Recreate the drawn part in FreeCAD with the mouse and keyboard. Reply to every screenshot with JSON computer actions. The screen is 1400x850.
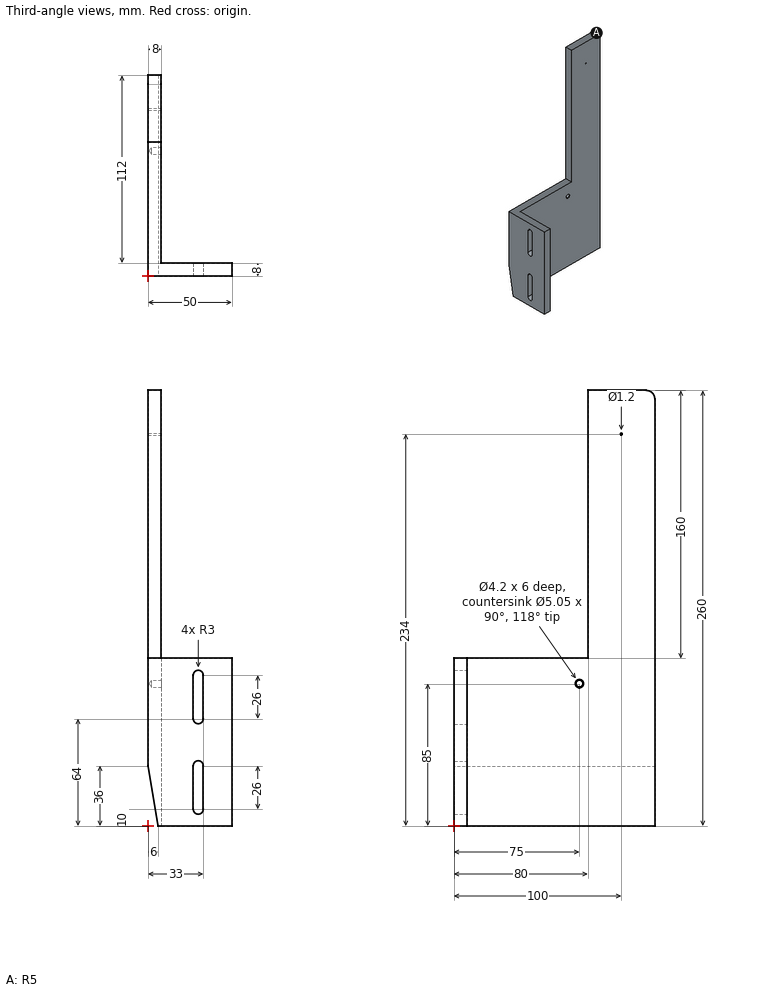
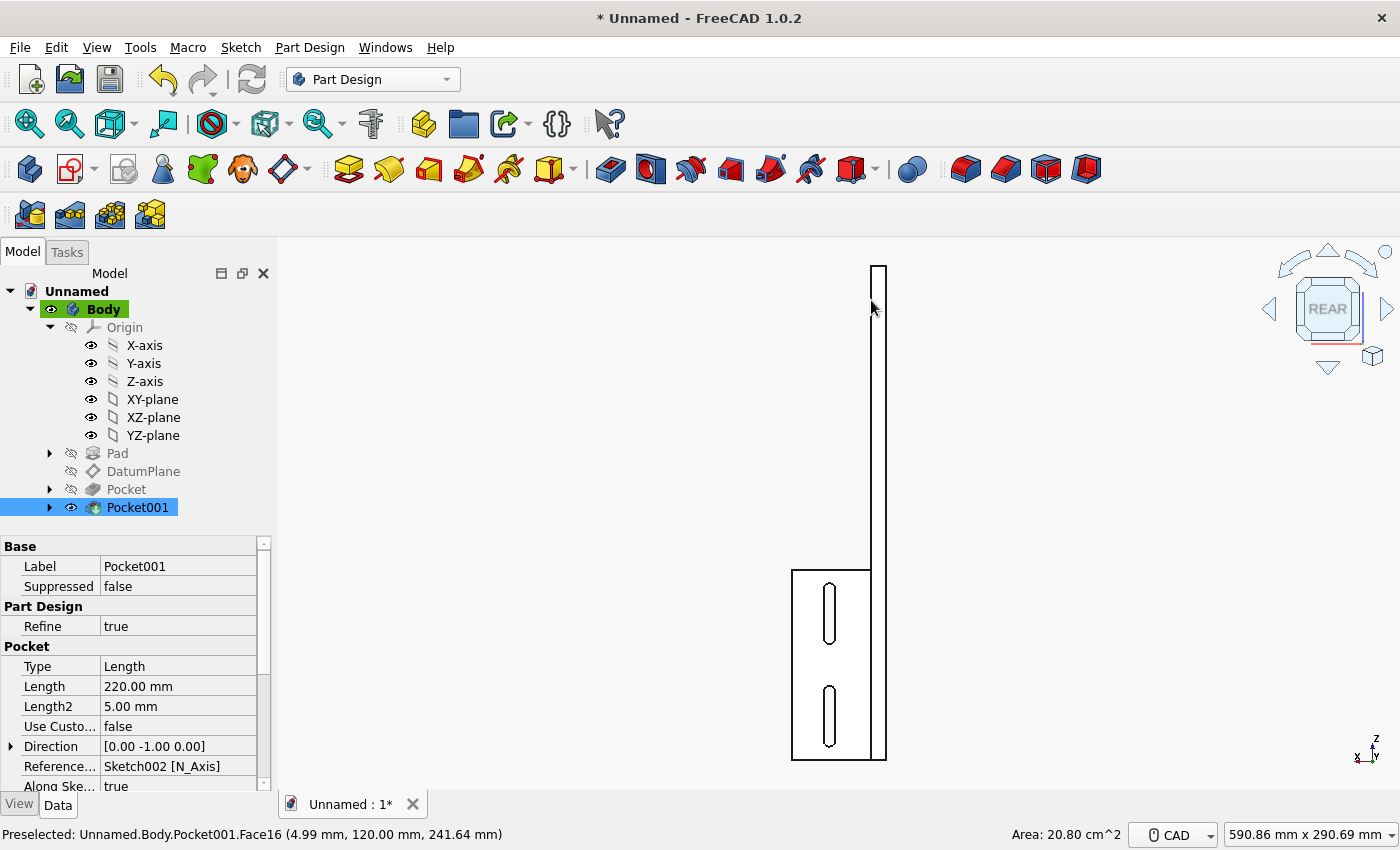
{"action": "left_click", "coordinate": [70, 170]}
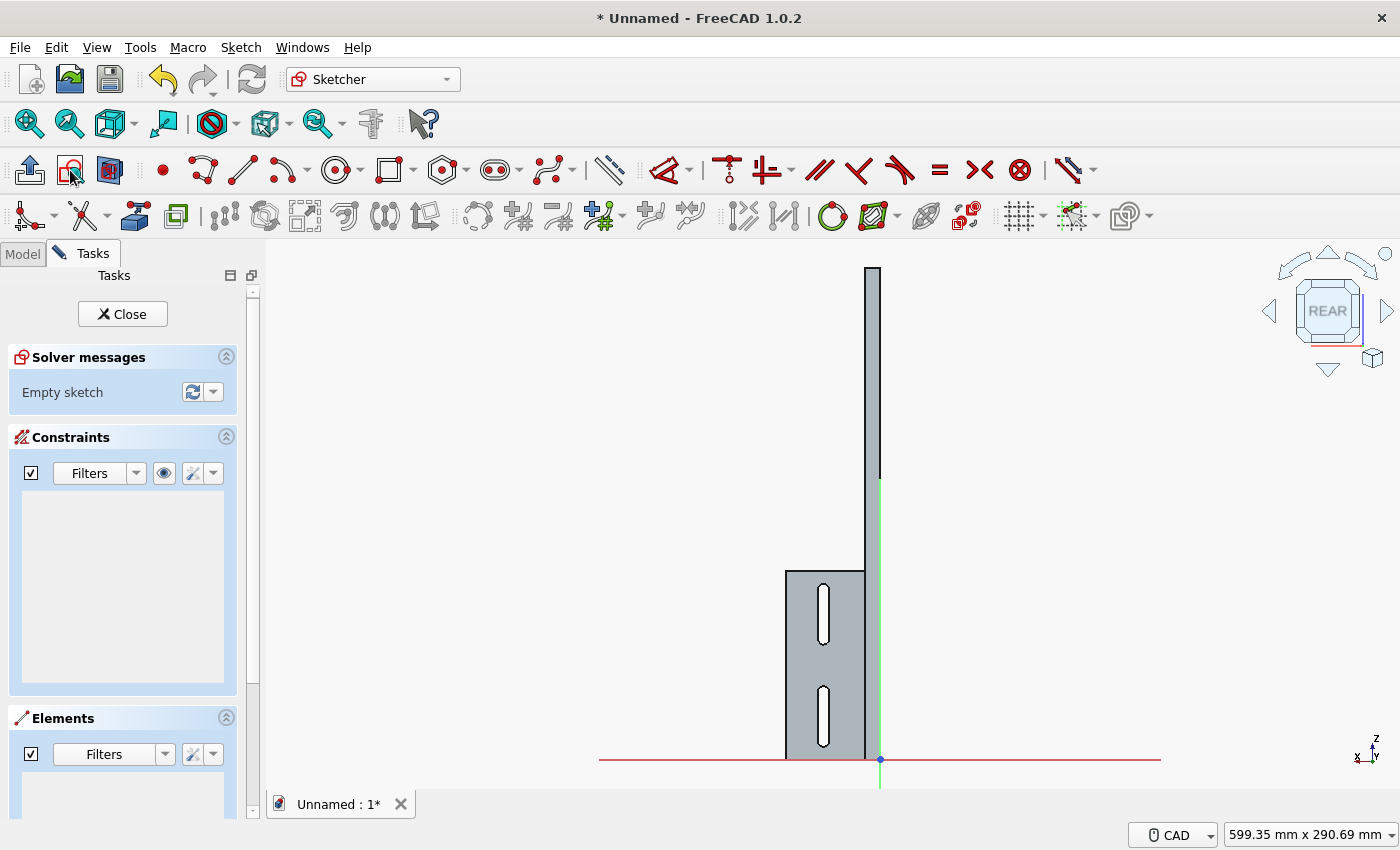
{"action": "scroll", "coordinate": [764, 514], "scroll_direction": "down", "scroll_amount": 5}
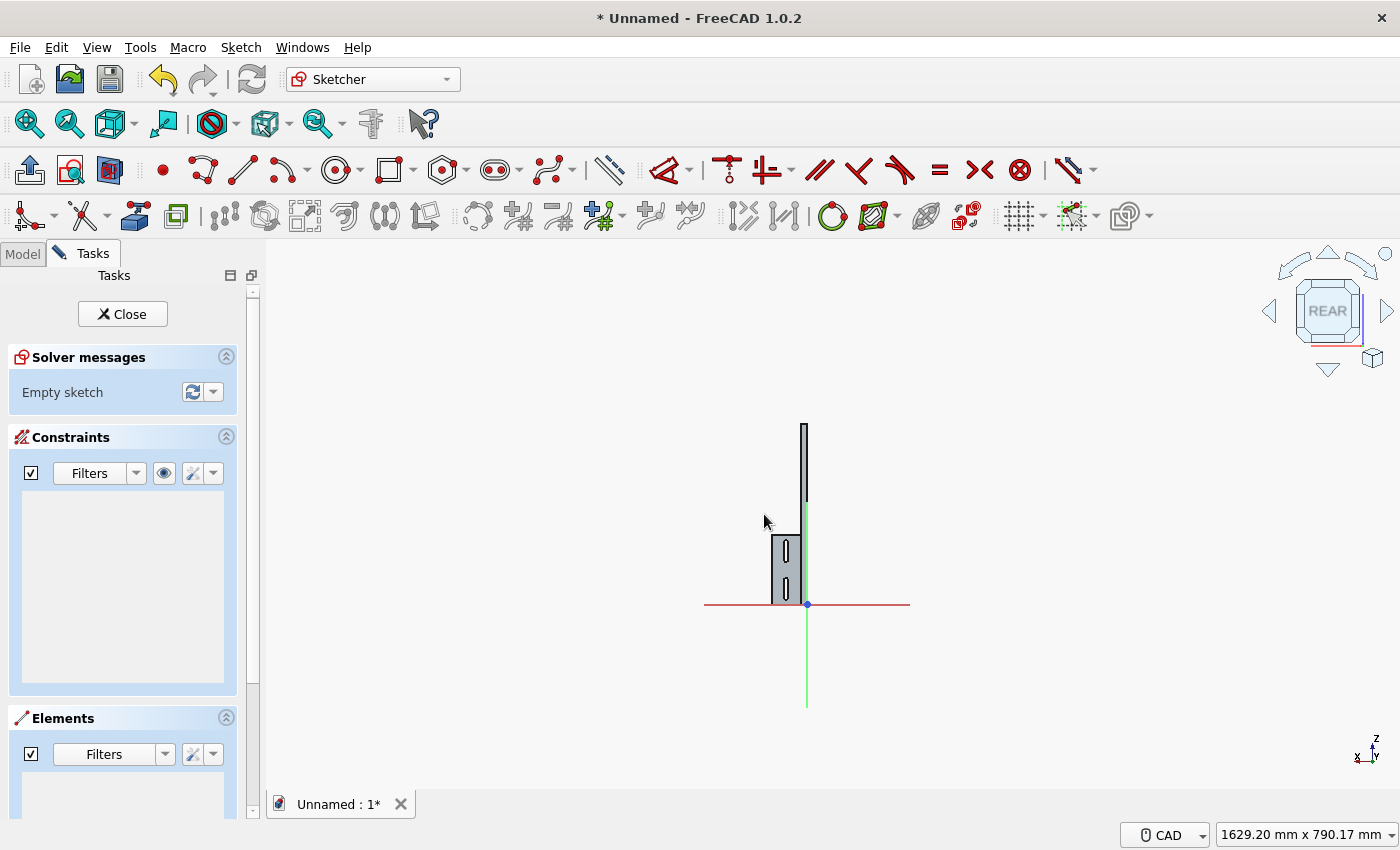
{"action": "scroll", "coordinate": [808, 599], "scroll_direction": "up", "scroll_amount": 13}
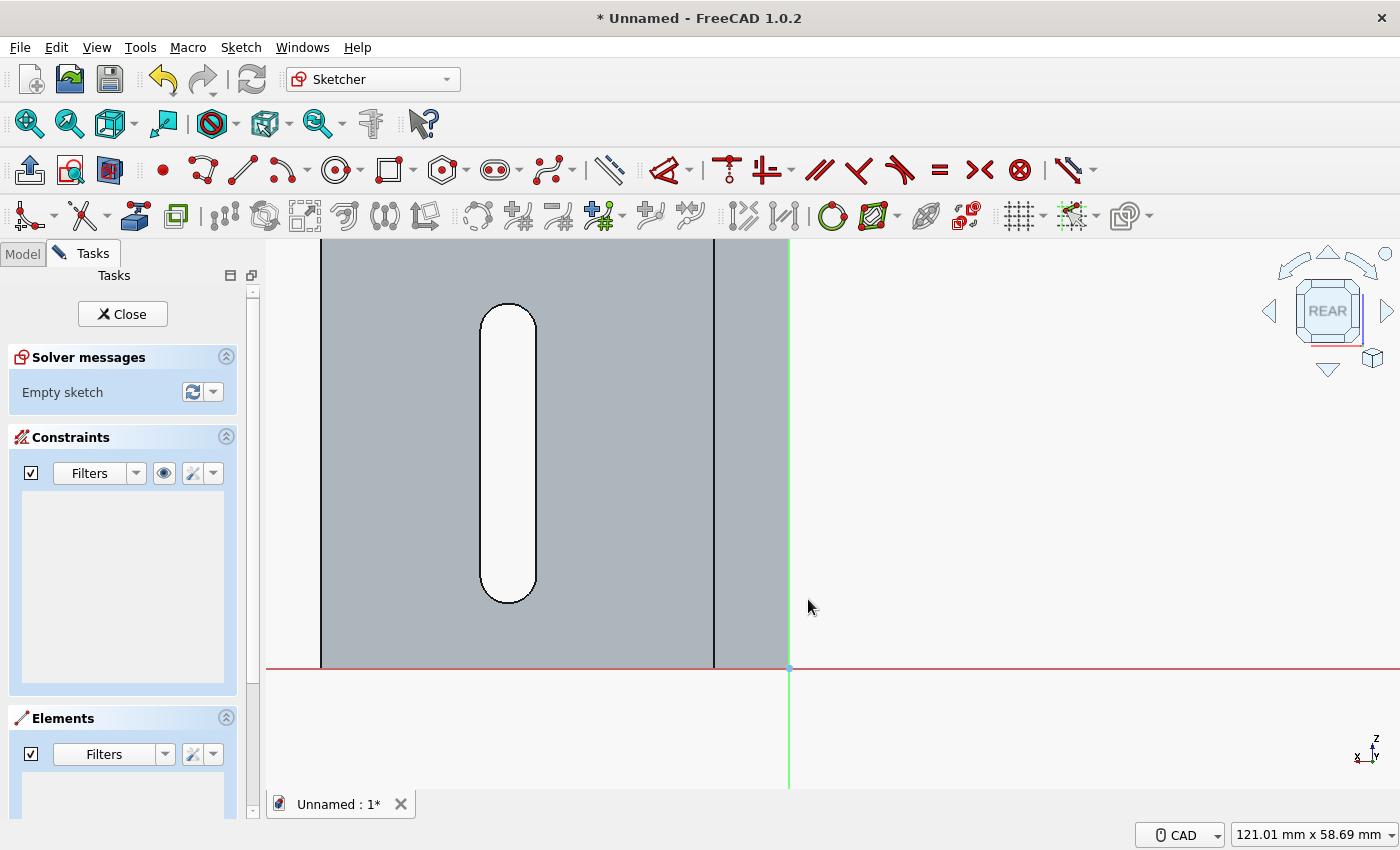
{"action": "left_click", "coordinate": [204, 170]}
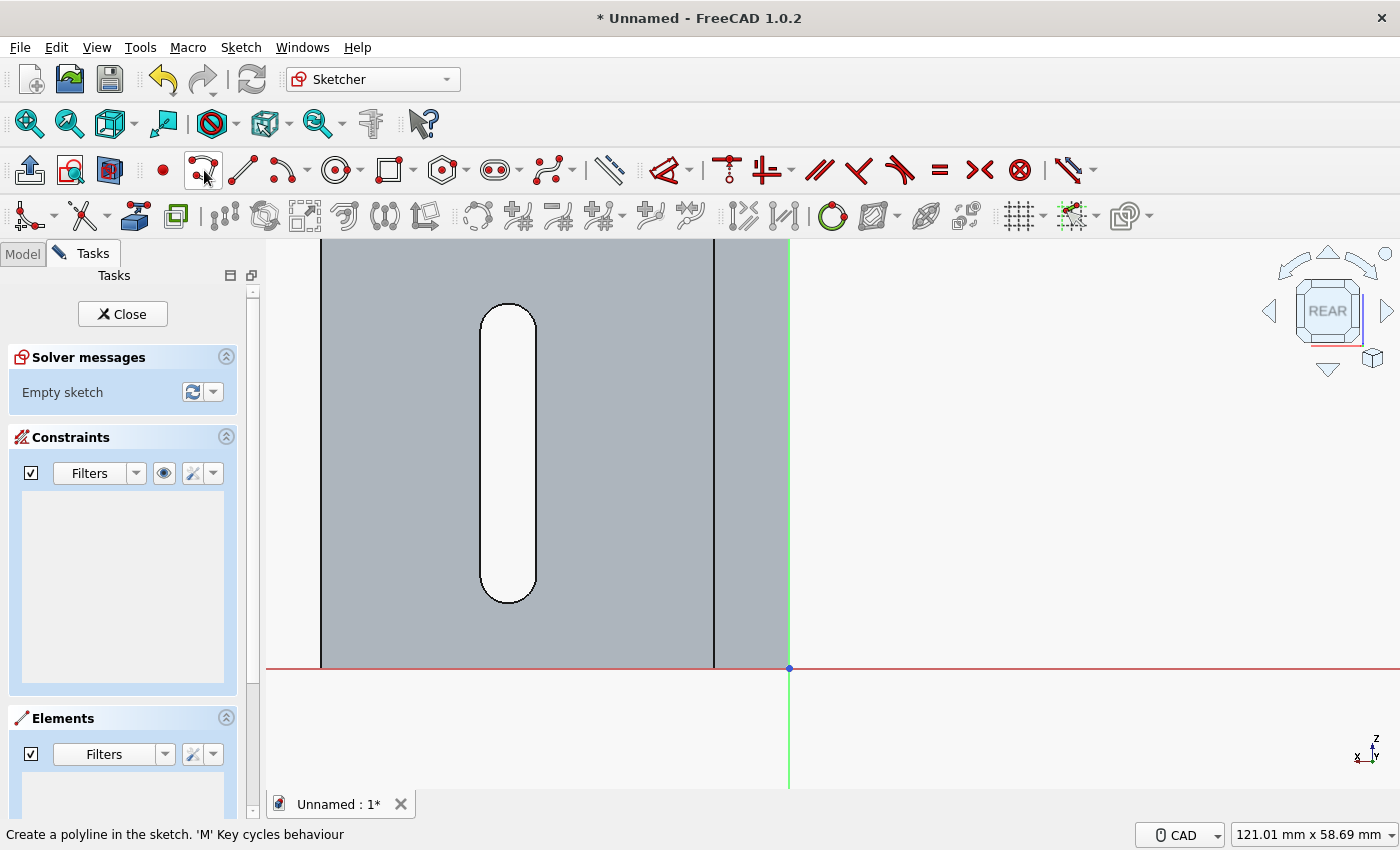
{"action": "left_click", "coordinate": [789, 669]}
{"action": "left_click", "coordinate": [780, 332]}
{"action": "left_click", "coordinate": [733, 660]}
{"action": "left_click", "coordinate": [789, 669]}
{"action": "key", "text": "Escape"}
{"action": "key", "text": "Escape"}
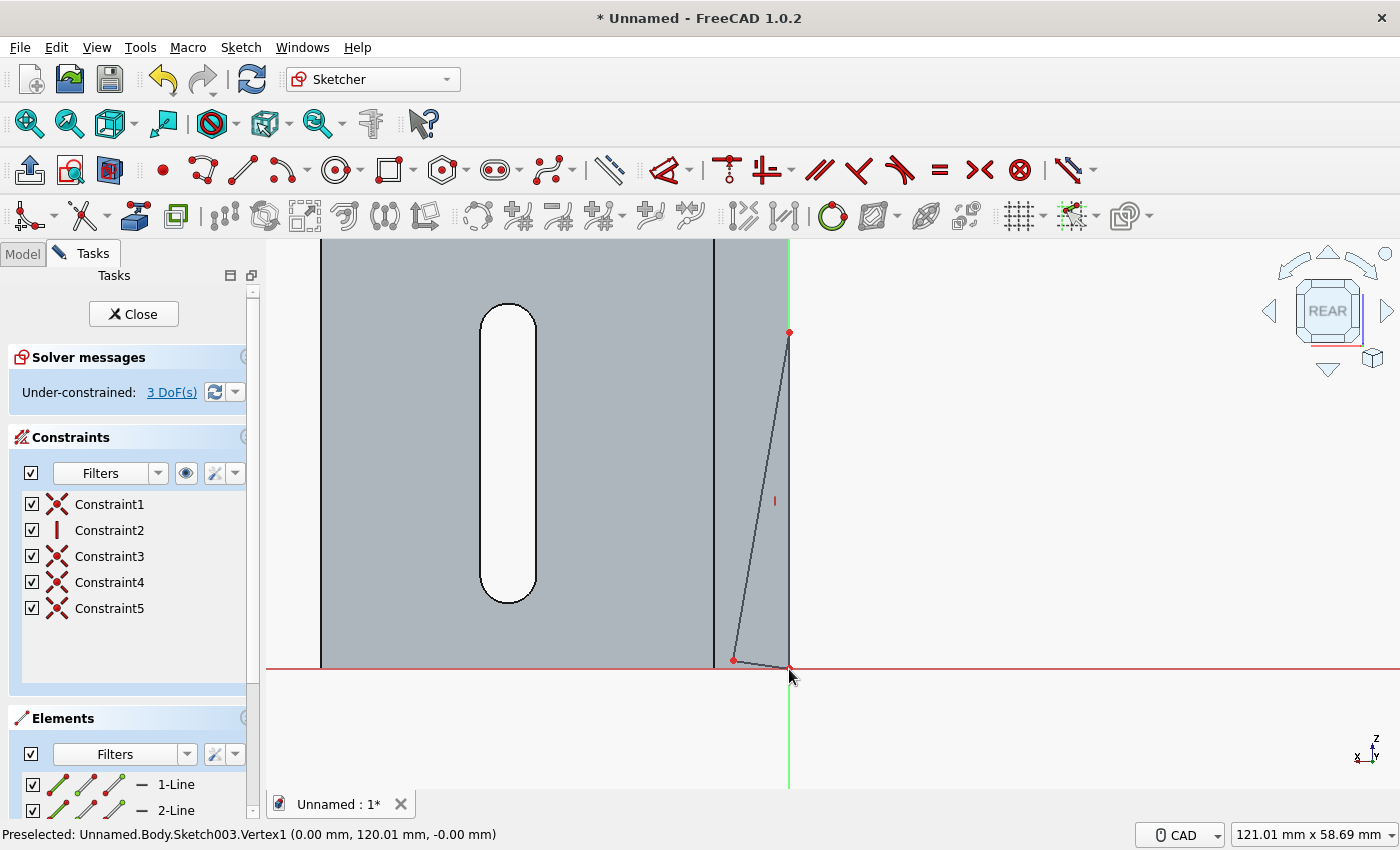
{"action": "left_click", "coordinate": [772, 667]}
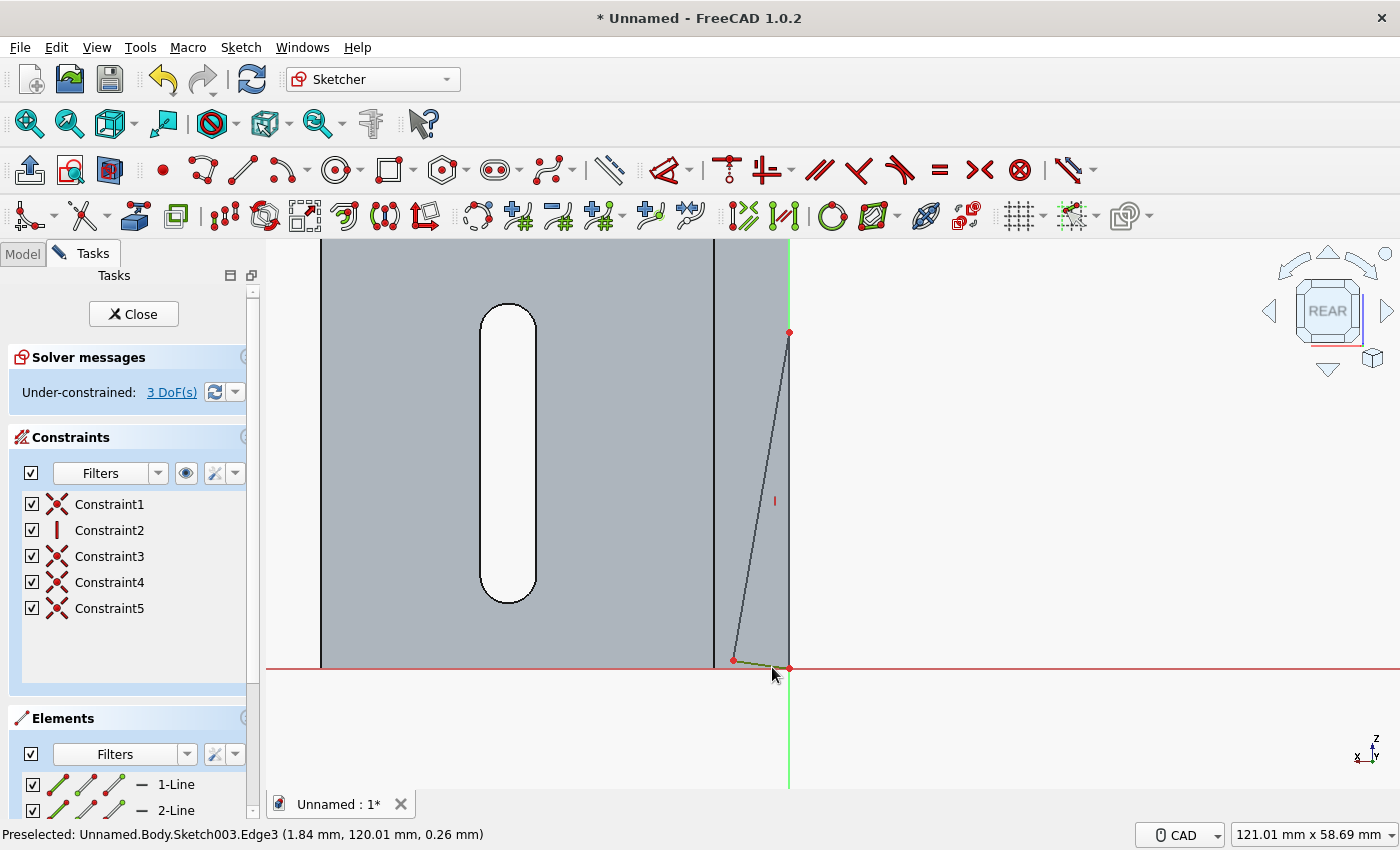
{"action": "left_click", "coordinate": [794, 170]}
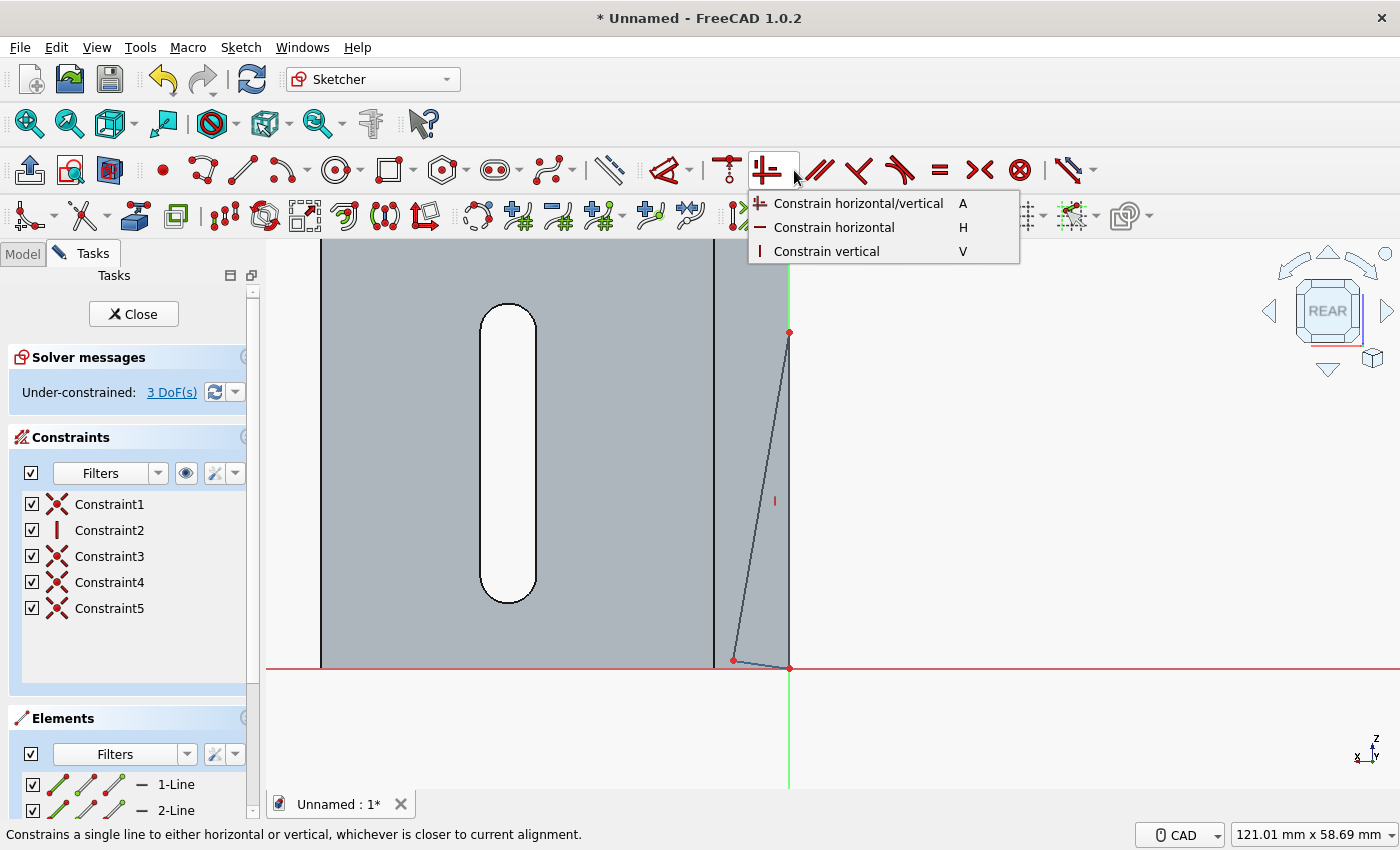
{"action": "left_click", "coordinate": [884, 227]}